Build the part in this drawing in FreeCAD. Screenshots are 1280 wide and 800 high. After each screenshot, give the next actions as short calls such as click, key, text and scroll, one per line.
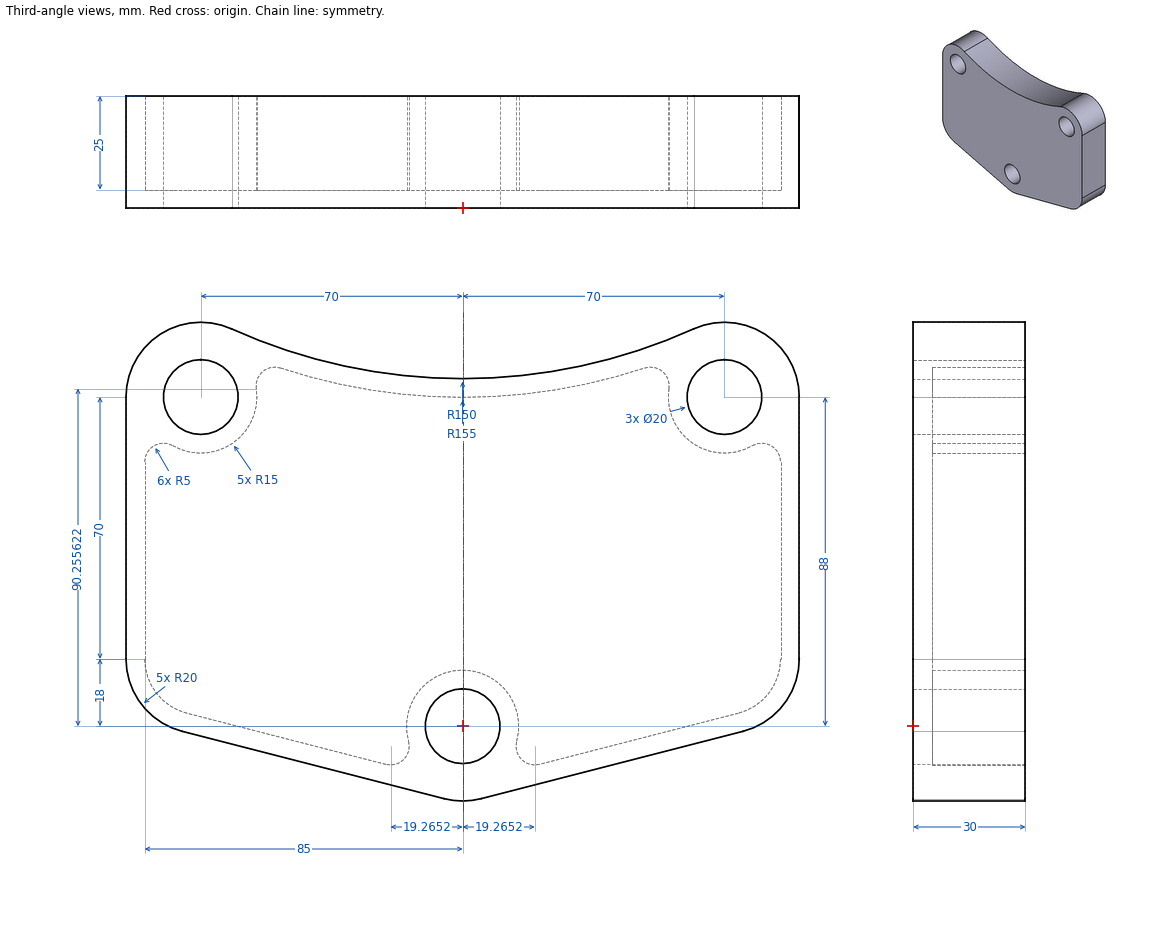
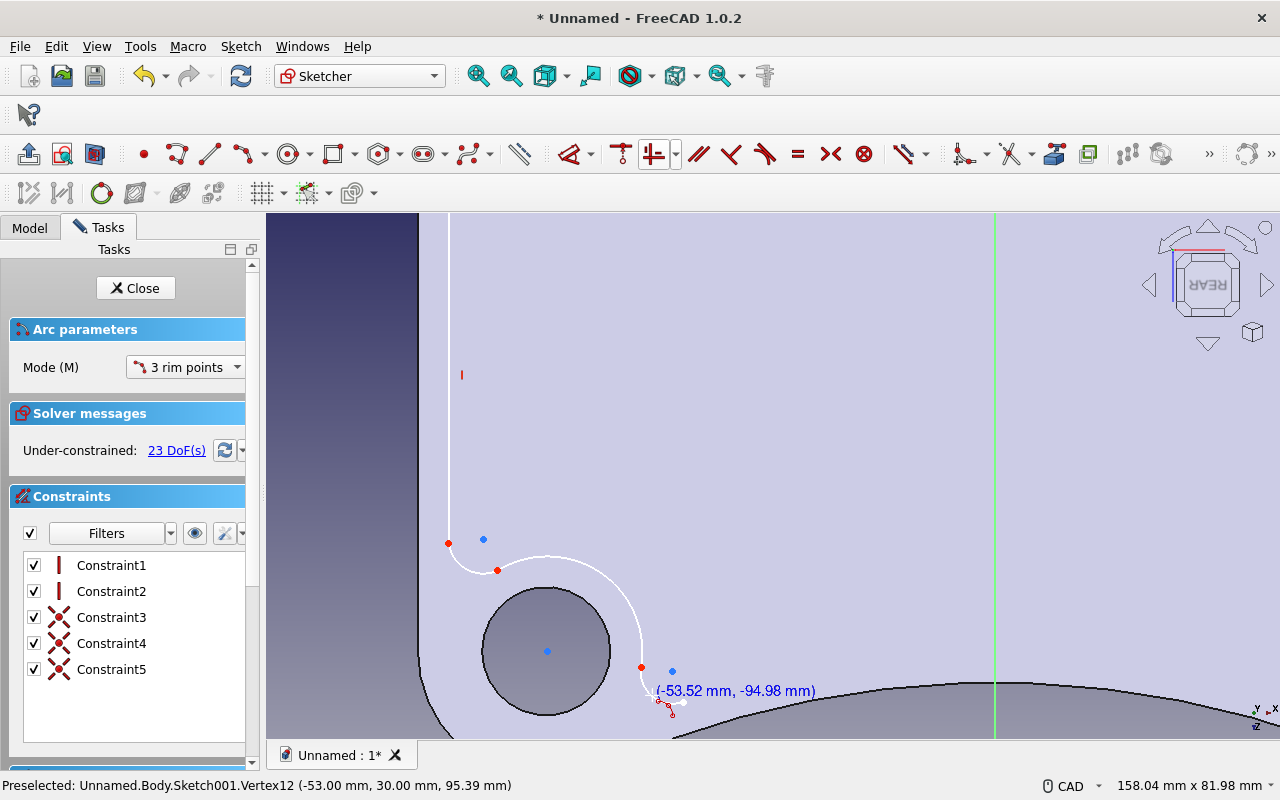
click(683, 702)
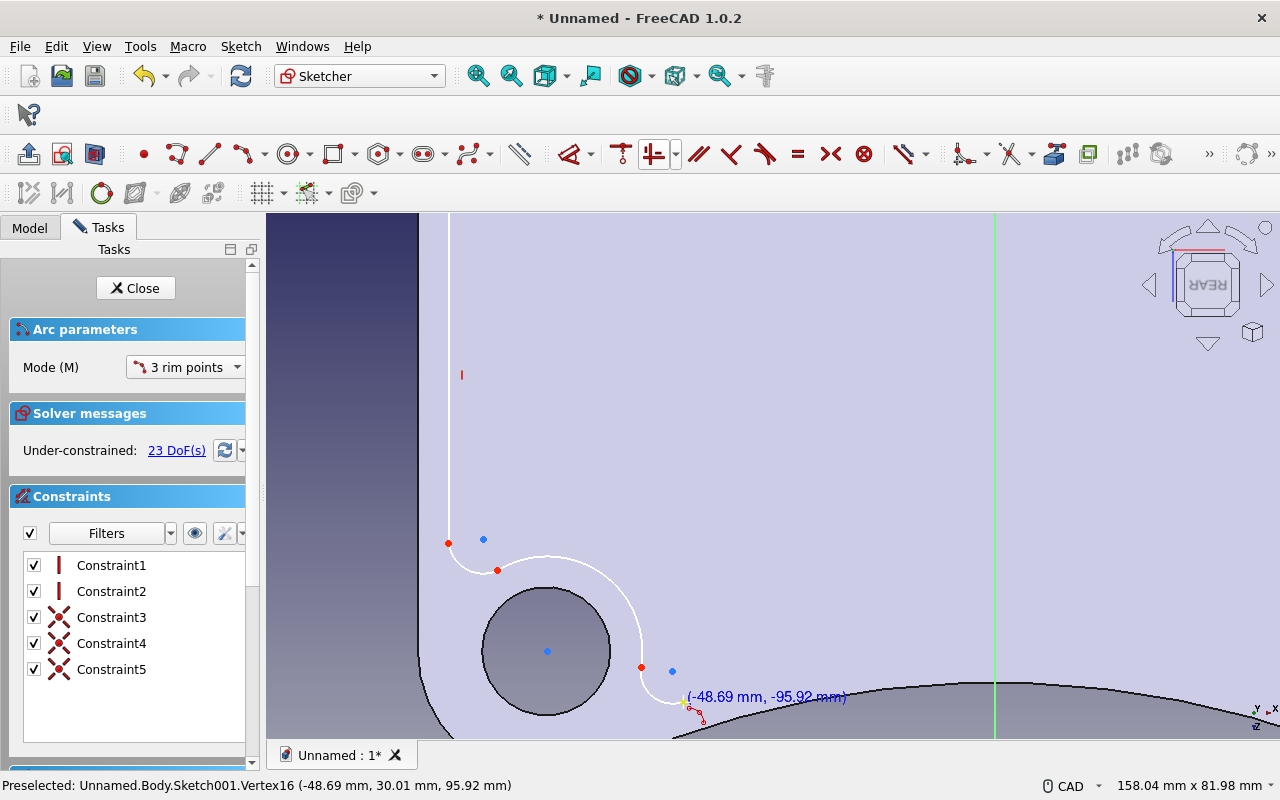
scroll(467, 570, down, 4)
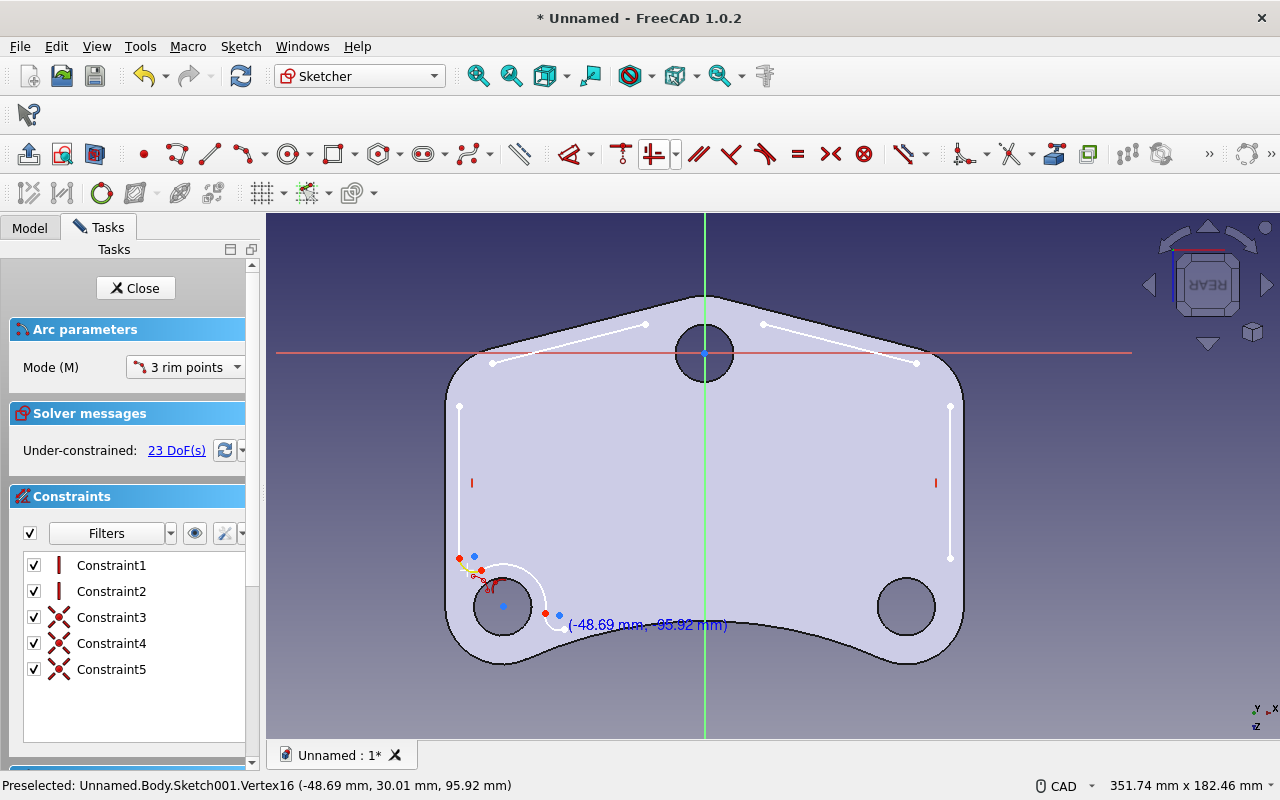
click(845, 629)
click(733, 608)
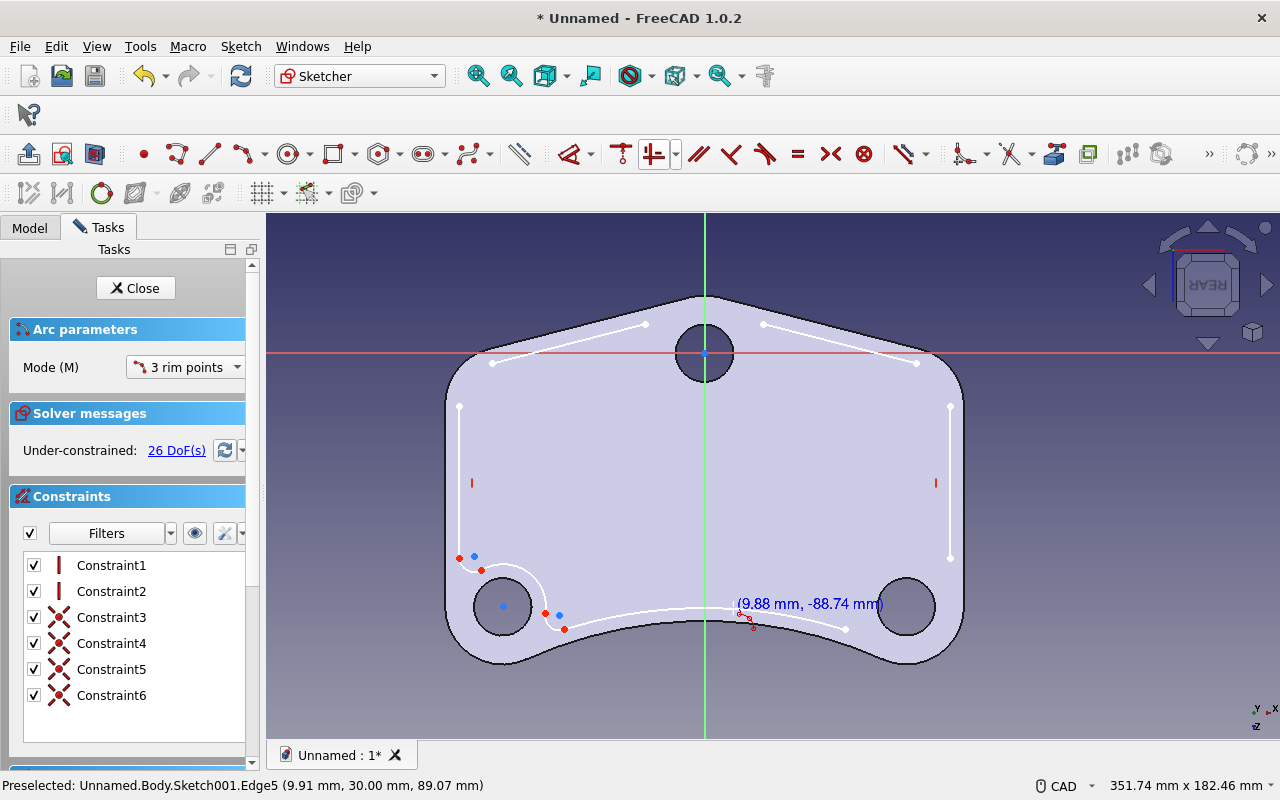
click(845, 630)
click(864, 613)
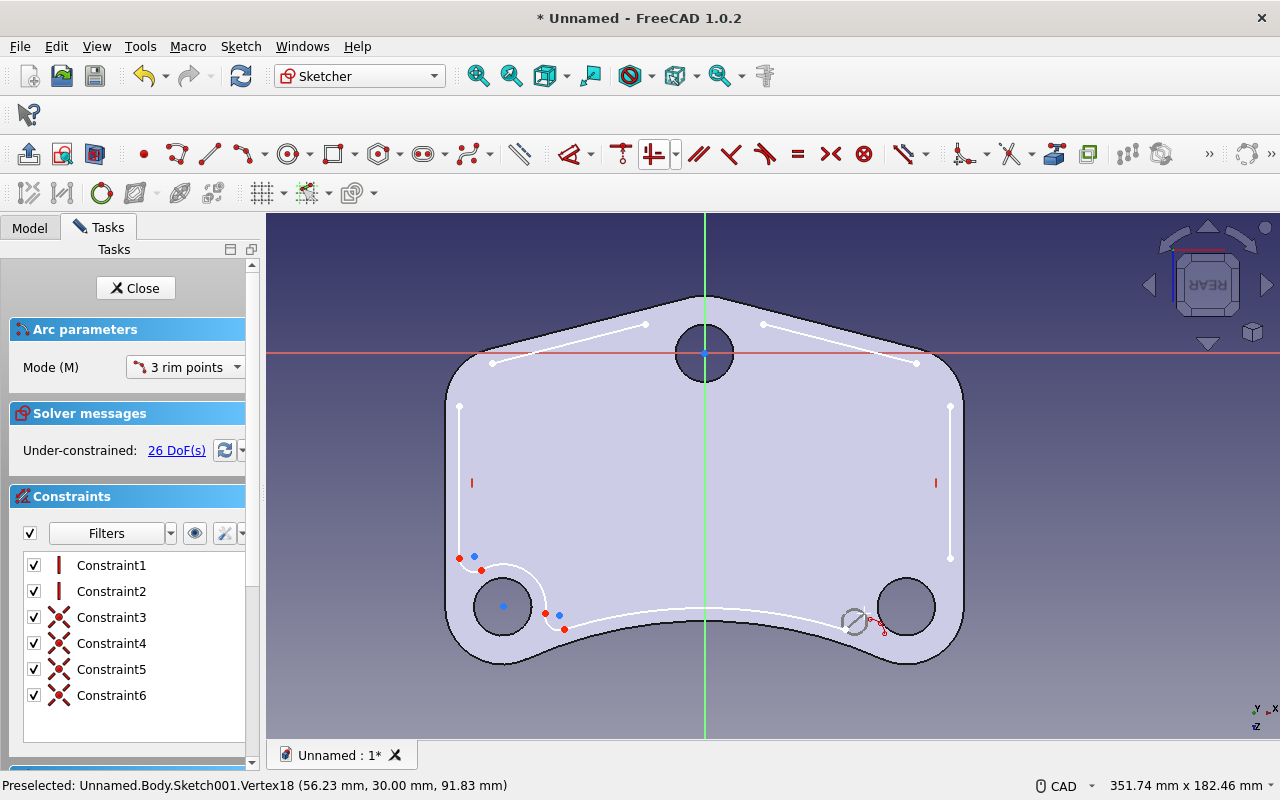
scroll(859, 627, up, 5)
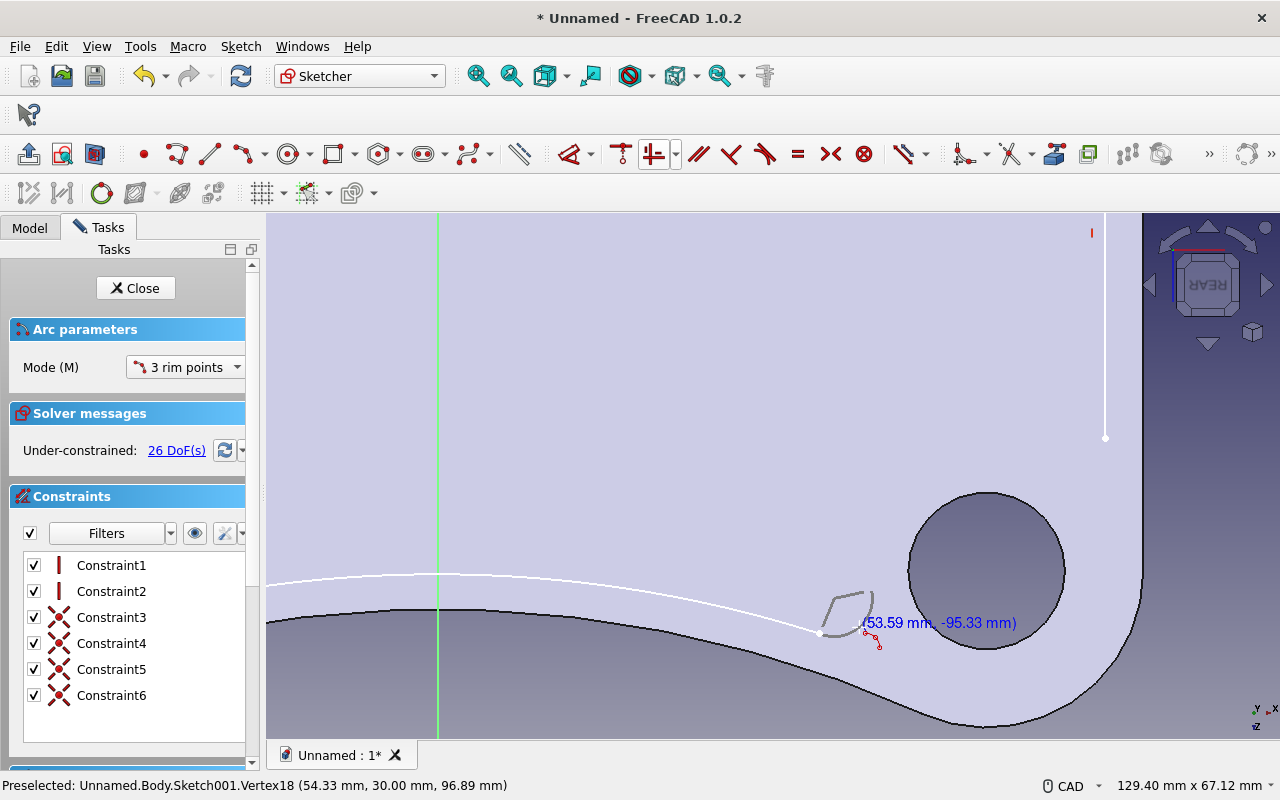
click(857, 624)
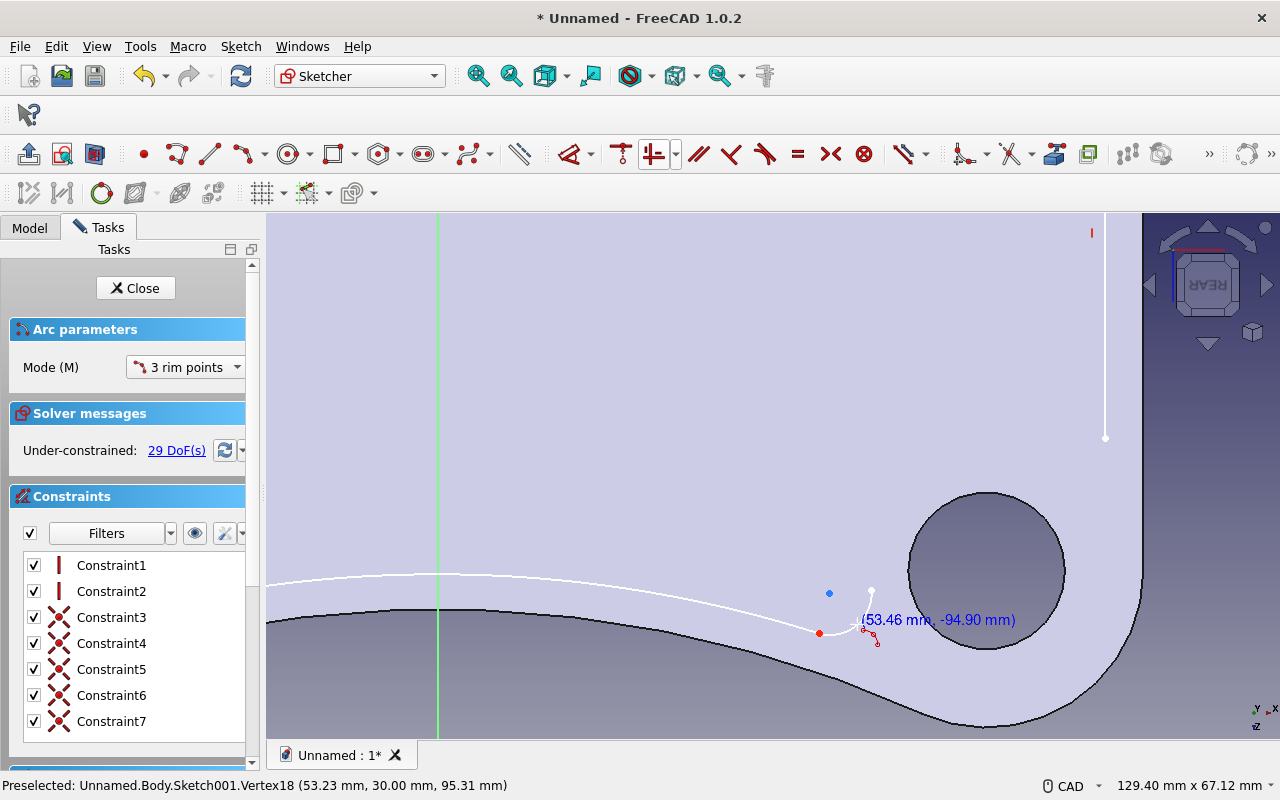
click(872, 590)
click(1045, 469)
click(920, 474)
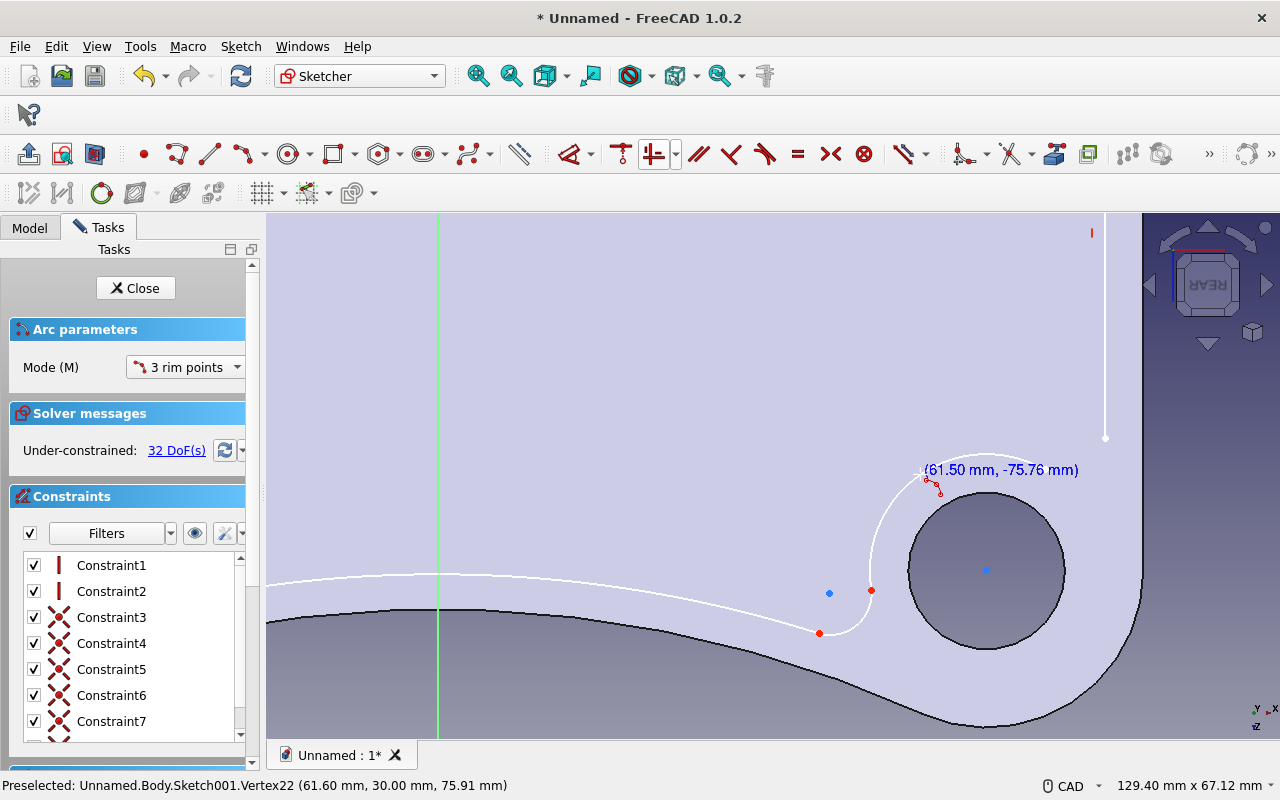
click(1045, 470)
click(1105, 439)
click(1085, 469)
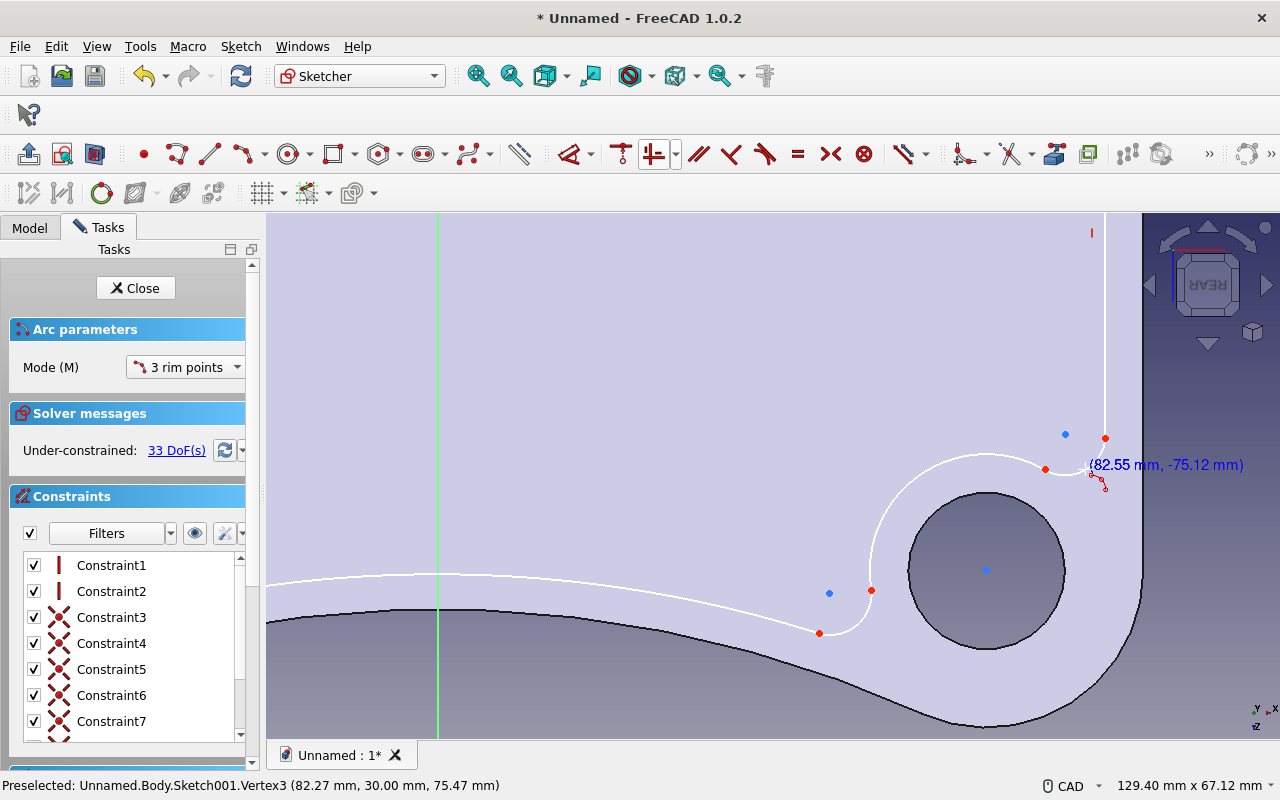
scroll(860, 627, down, 5)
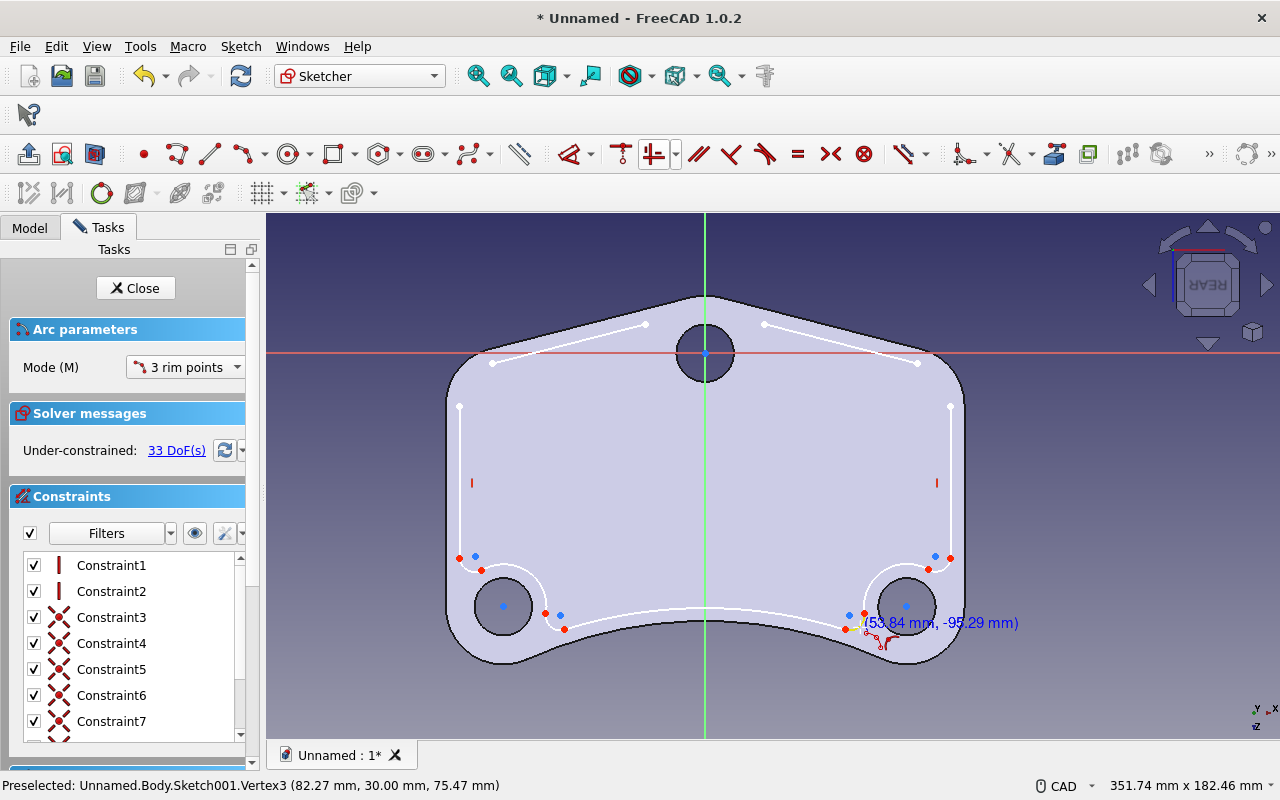
click(951, 407)